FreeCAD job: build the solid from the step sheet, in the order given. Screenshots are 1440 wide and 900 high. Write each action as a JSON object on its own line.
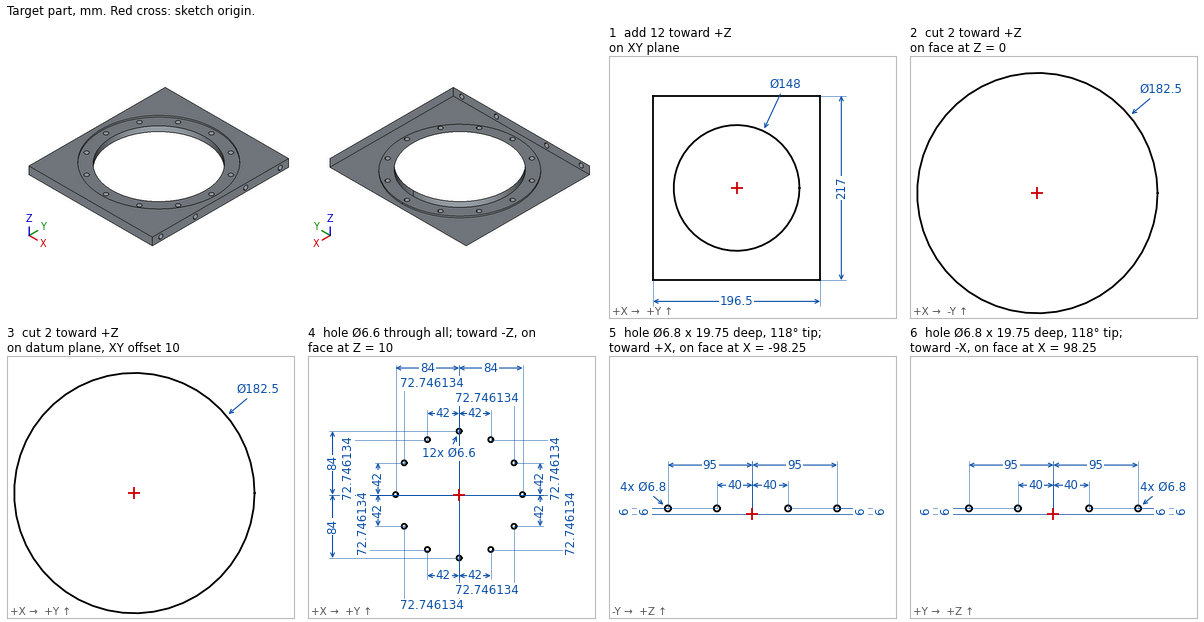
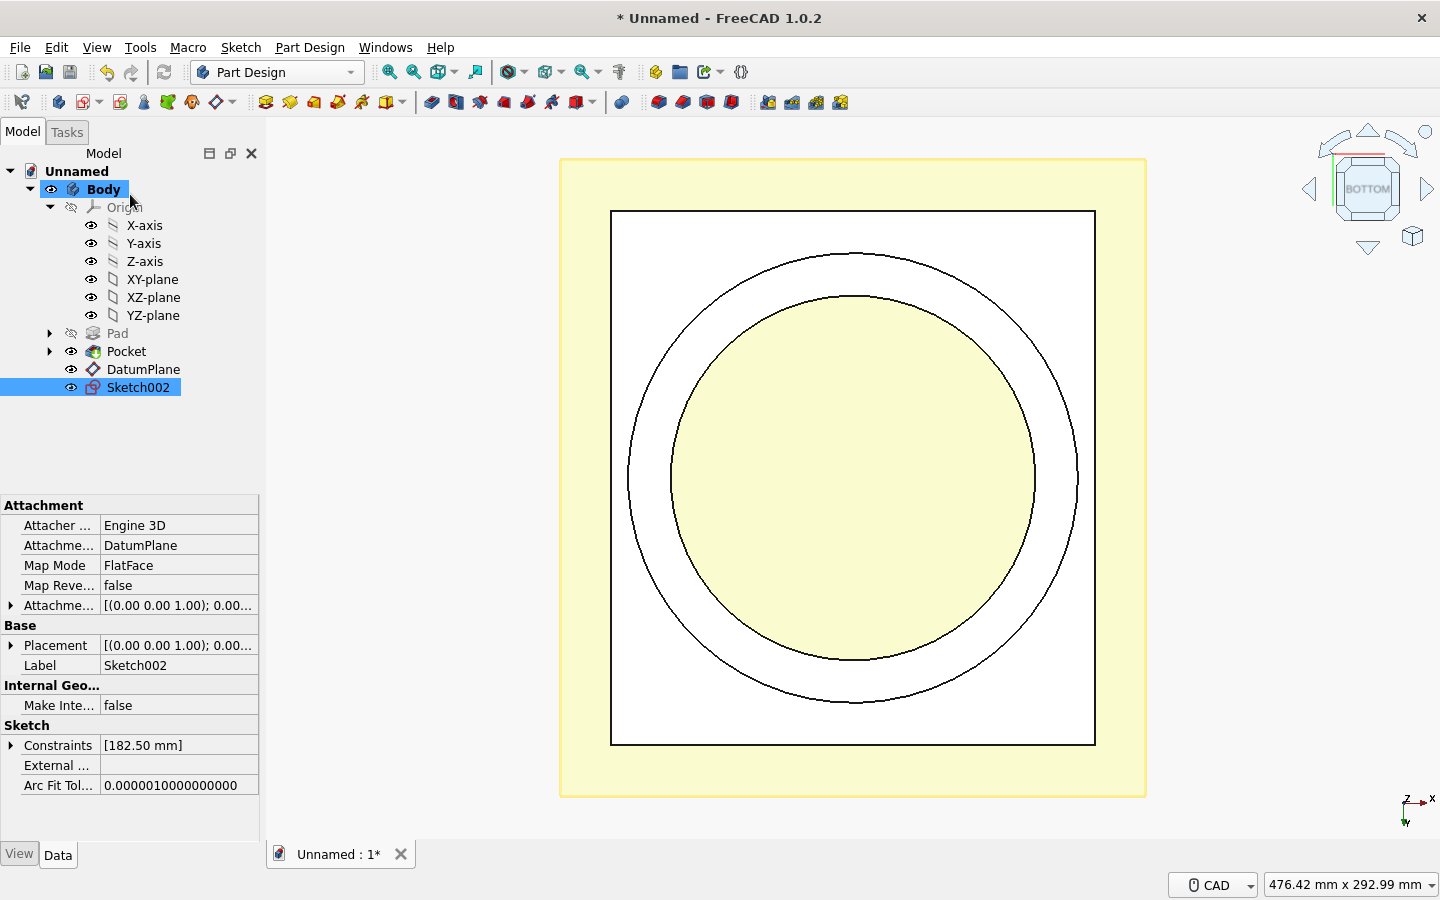
{"action": "left_click", "coordinate": [432, 102]}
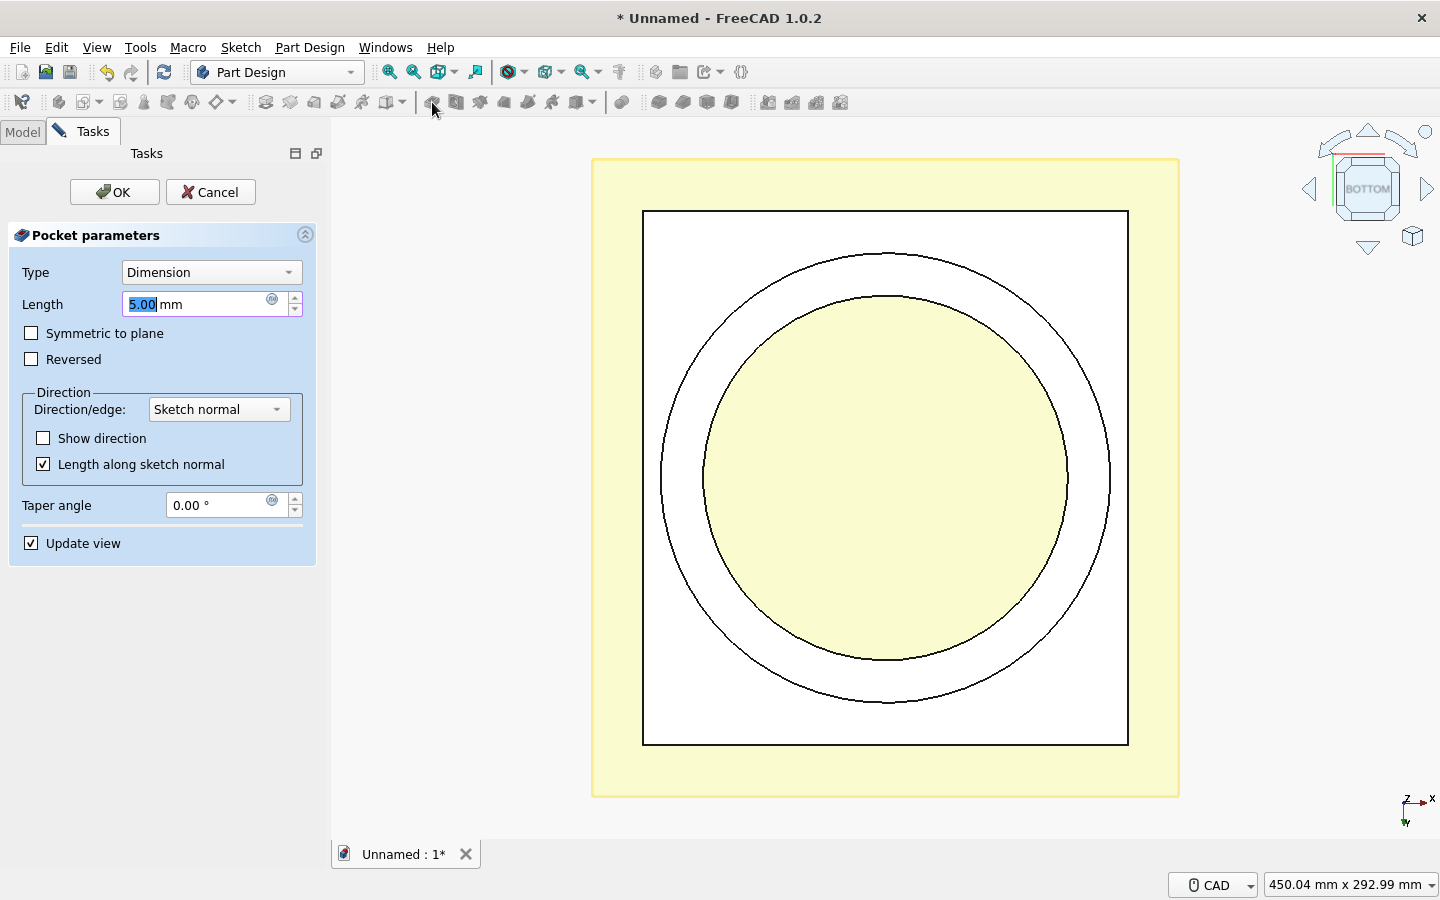
{"action": "type", "text": "2"}
{"action": "key", "text": "Tab"}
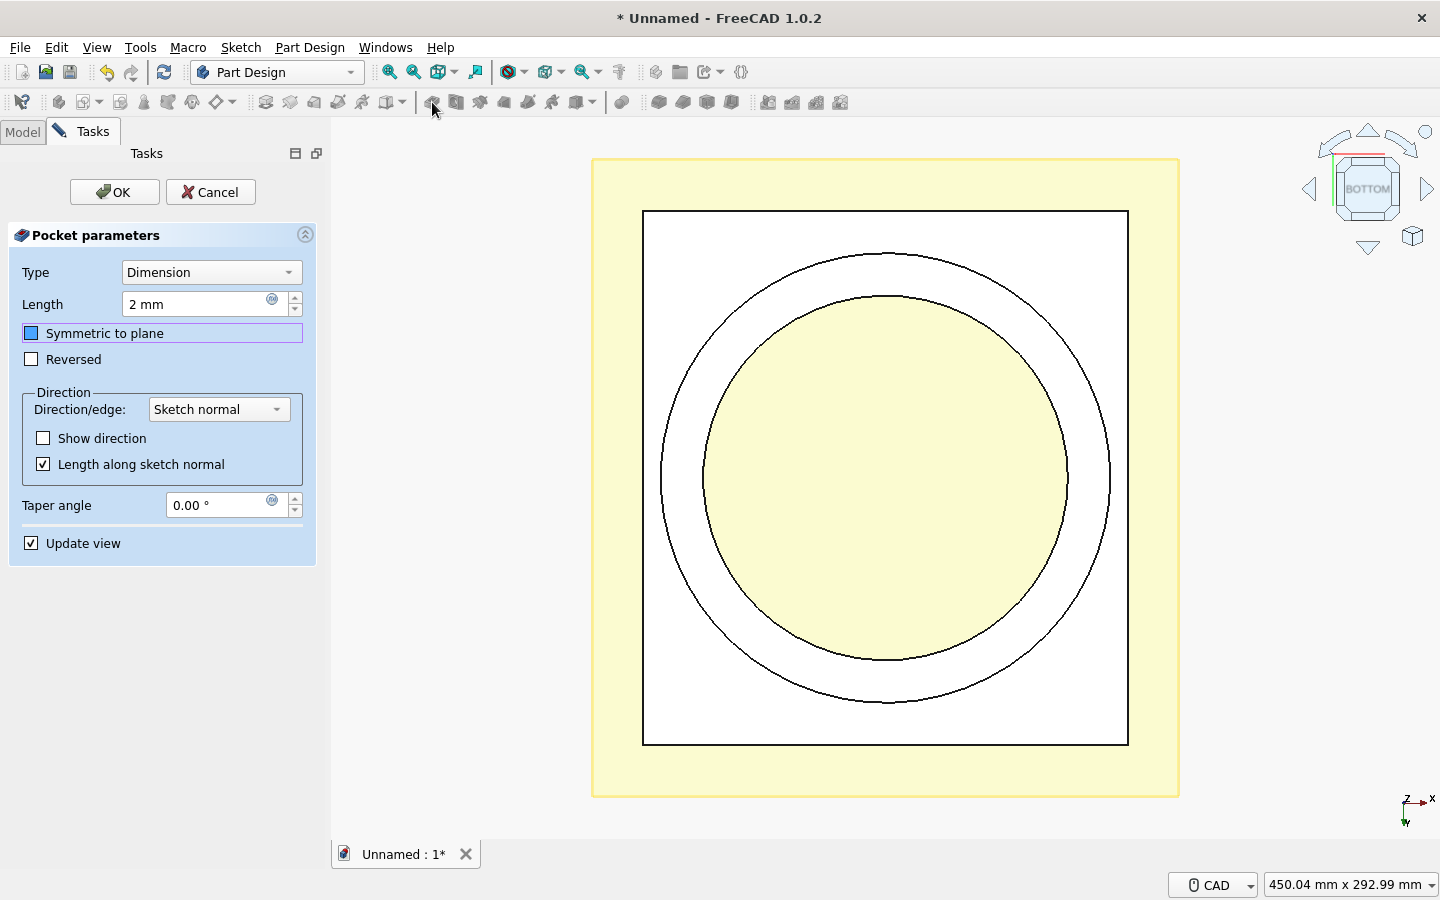
{"action": "left_click", "coordinate": [30, 359]}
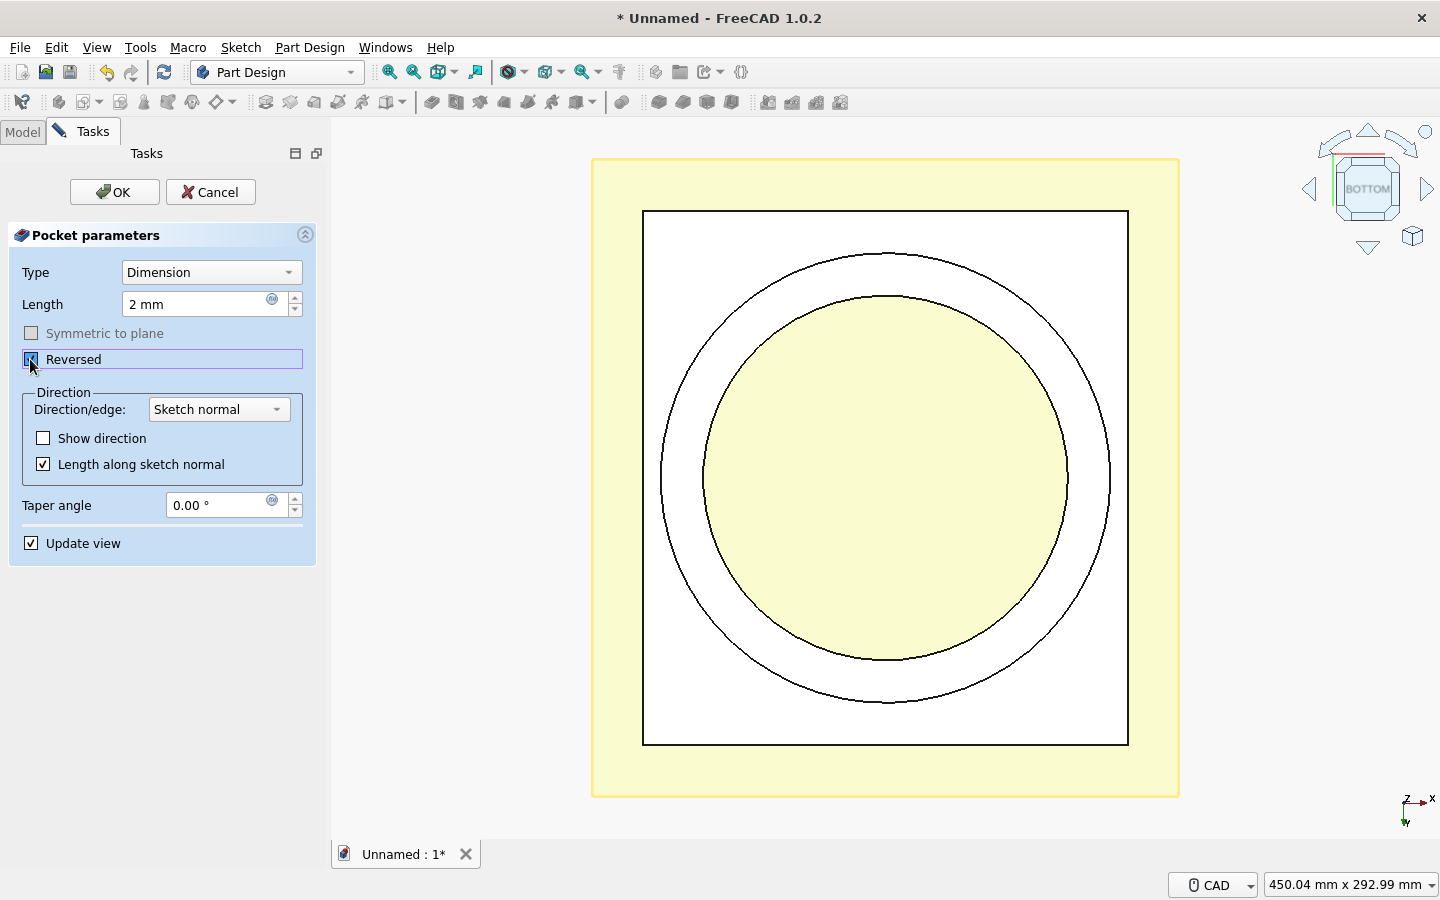
{"action": "left_click", "coordinate": [115, 192]}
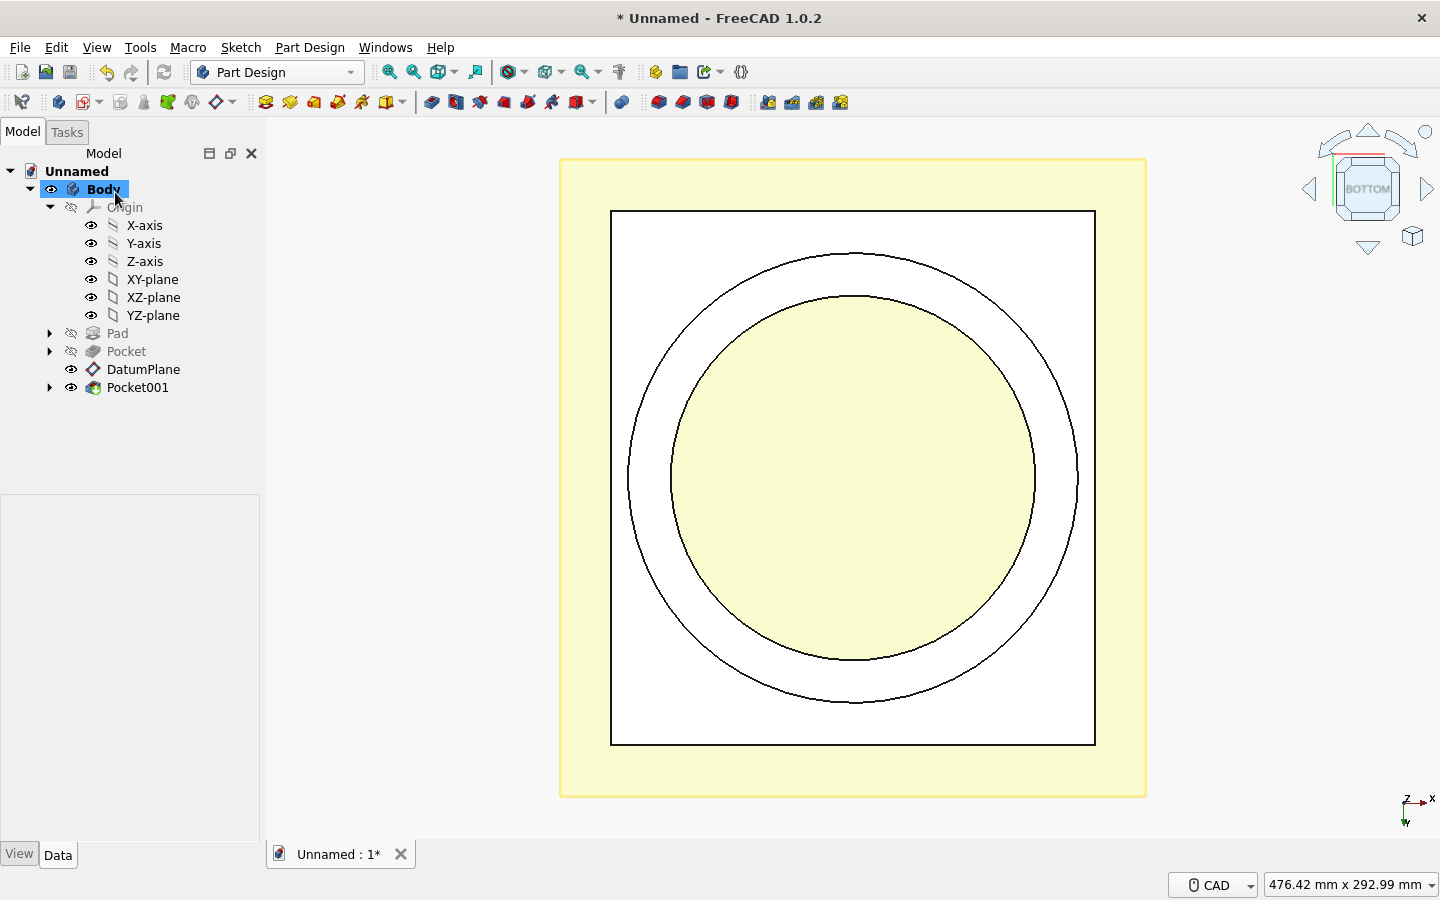
{"action": "left_click", "coordinate": [116, 369]}
{"action": "key", "text": "space"}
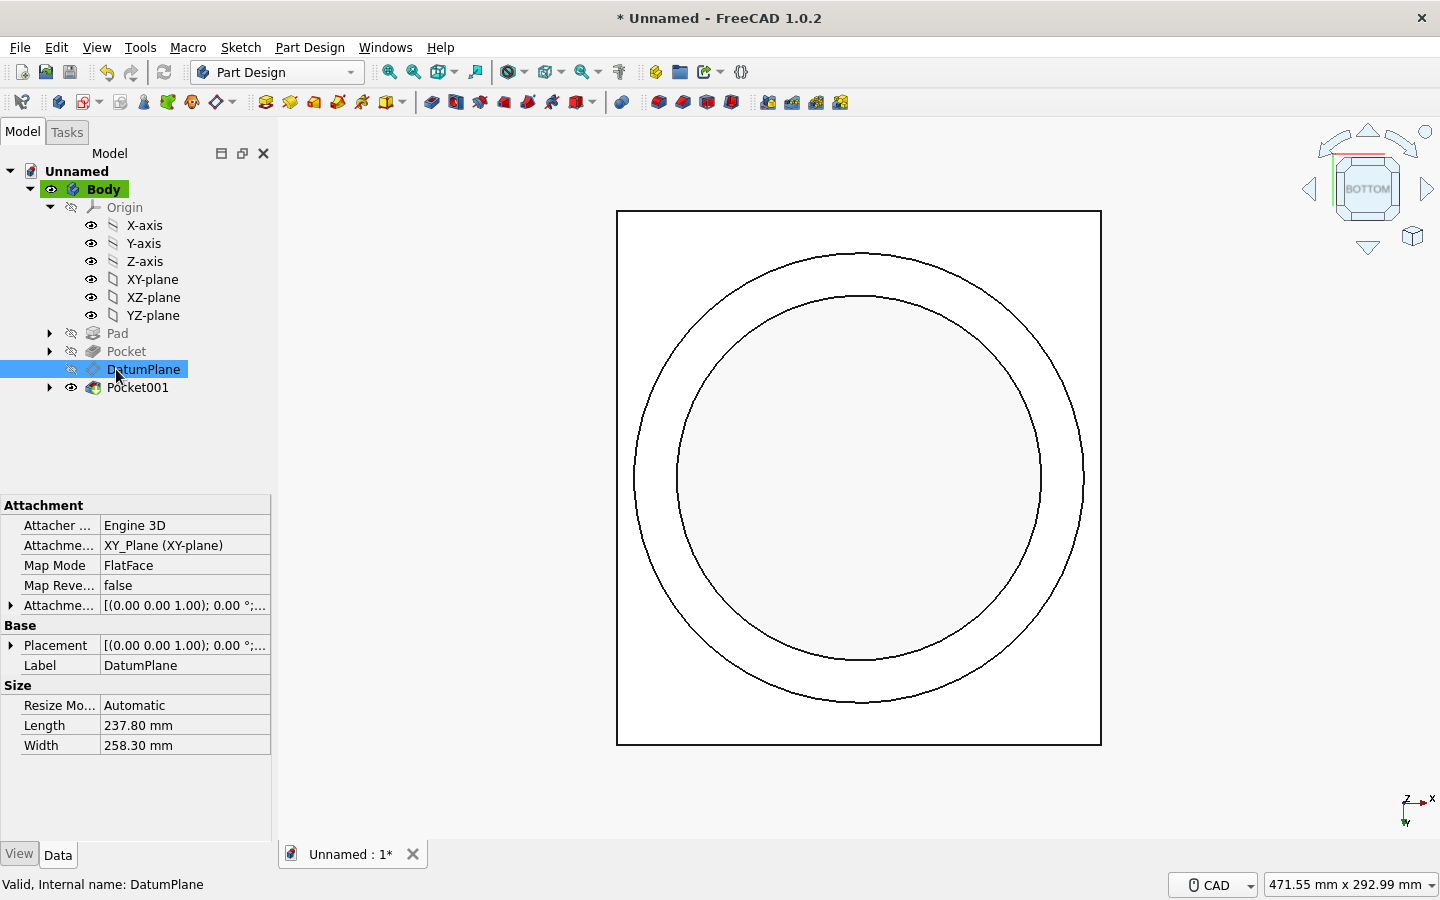
{"action": "key", "text": "0"}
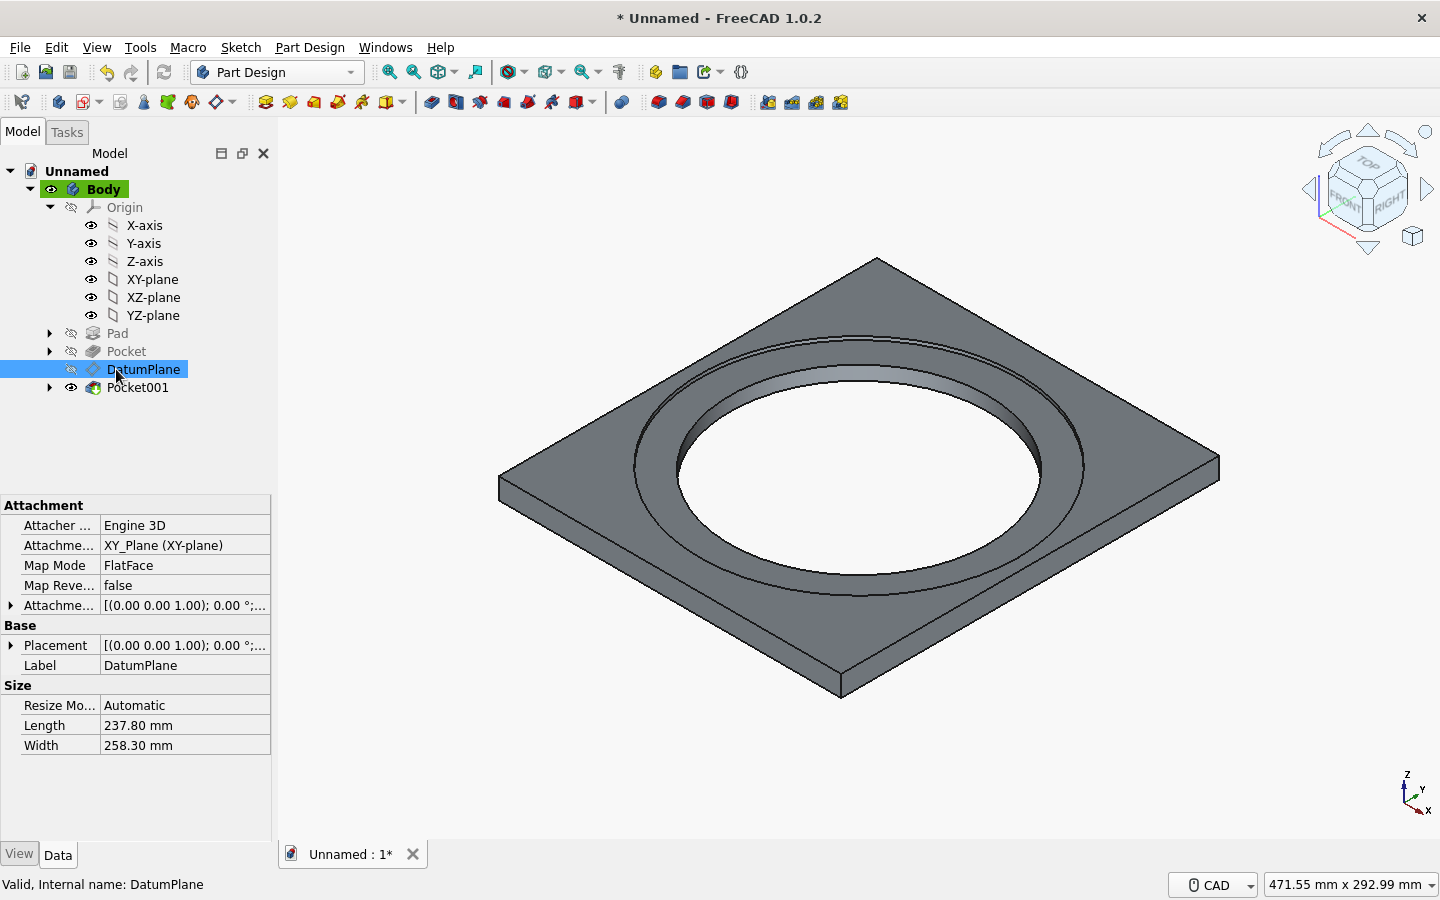
{"action": "left_click", "coordinate": [1041, 416]}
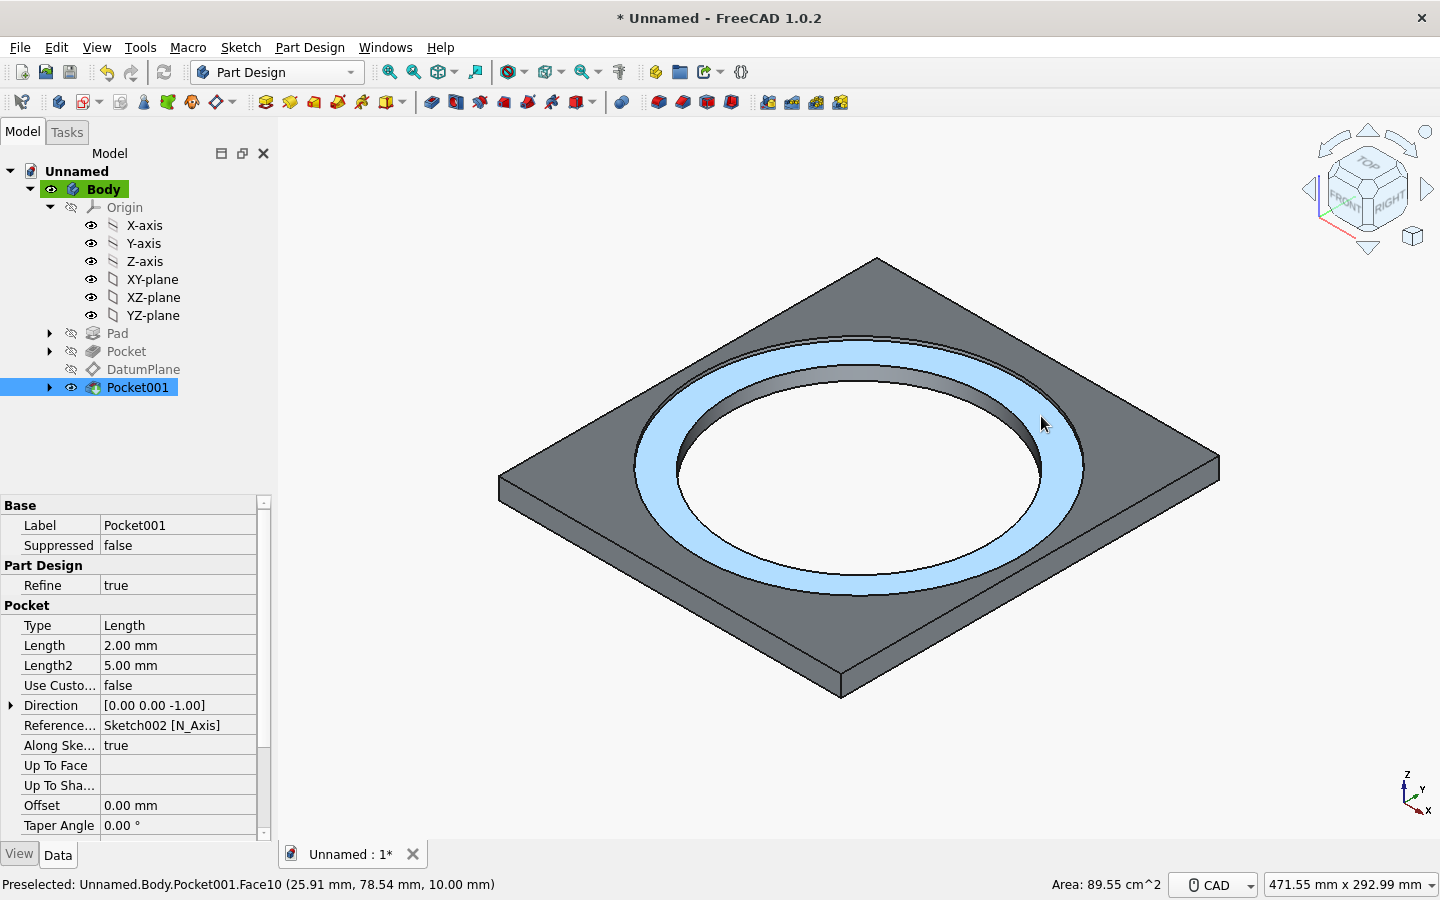
{"action": "left_click", "coordinate": [84, 102]}